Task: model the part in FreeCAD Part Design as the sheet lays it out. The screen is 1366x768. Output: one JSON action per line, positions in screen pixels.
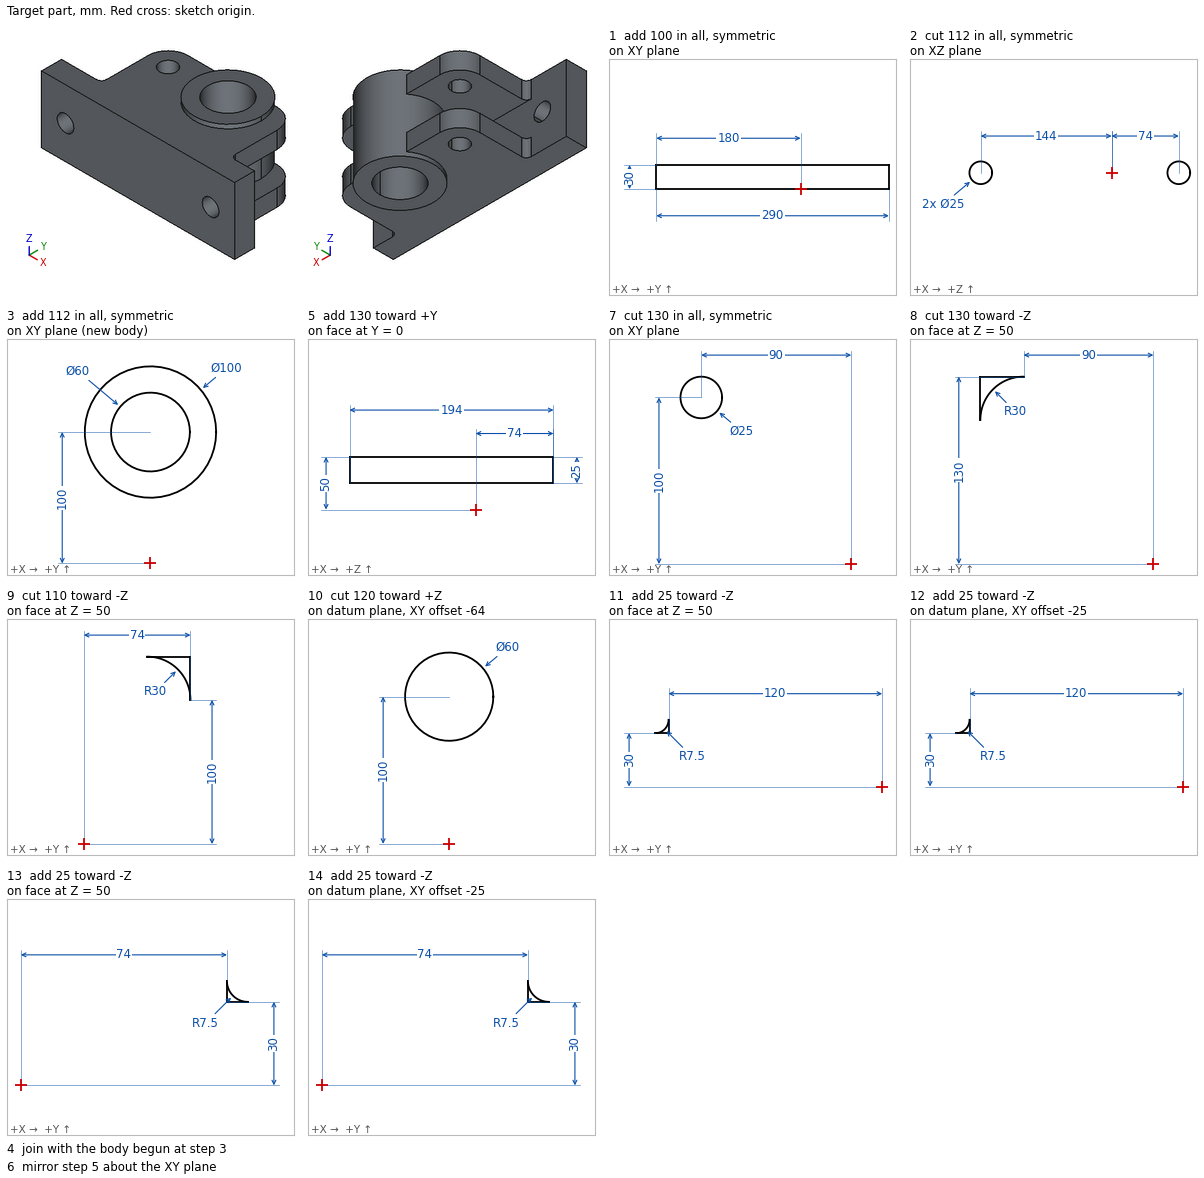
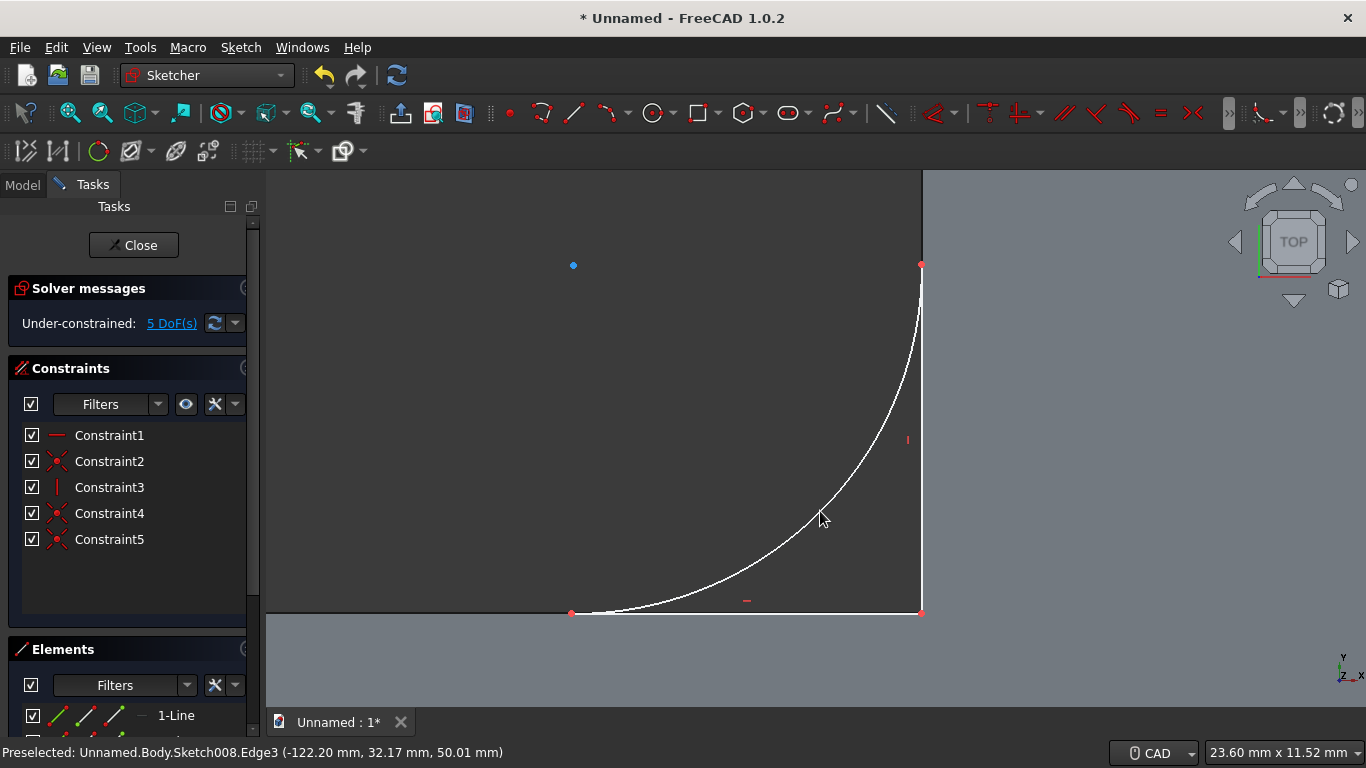
{"action": "left_click", "coordinate": [677, 614]}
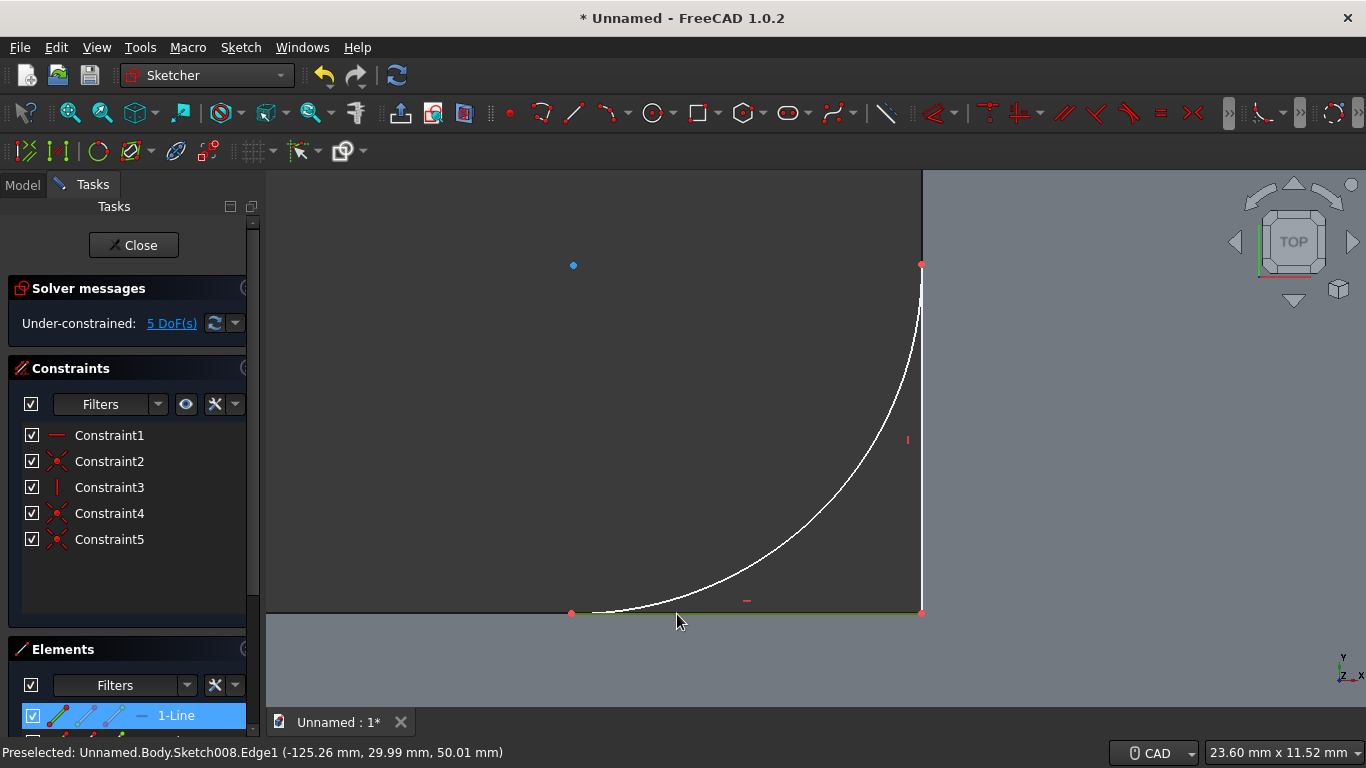
{"action": "left_click", "coordinate": [731, 576]}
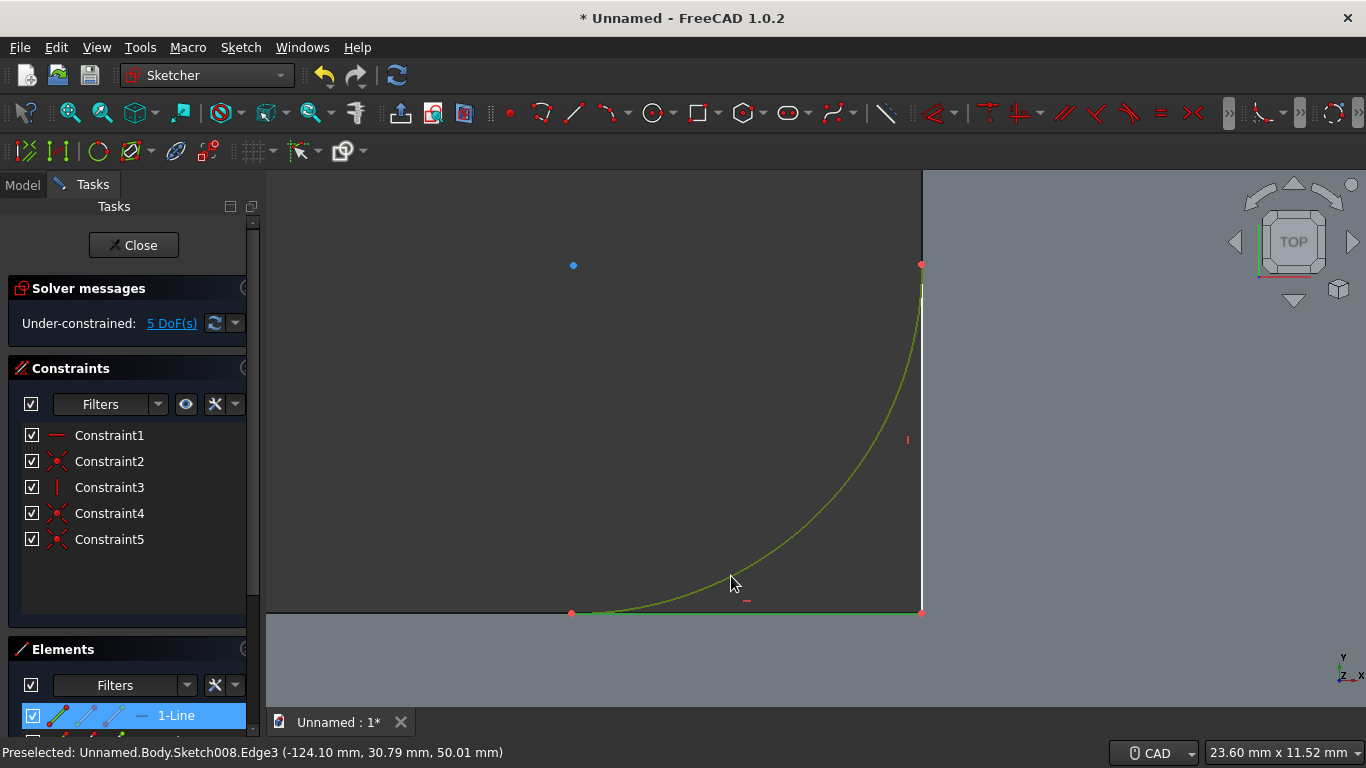
{"action": "left_click", "coordinate": [1130, 114]}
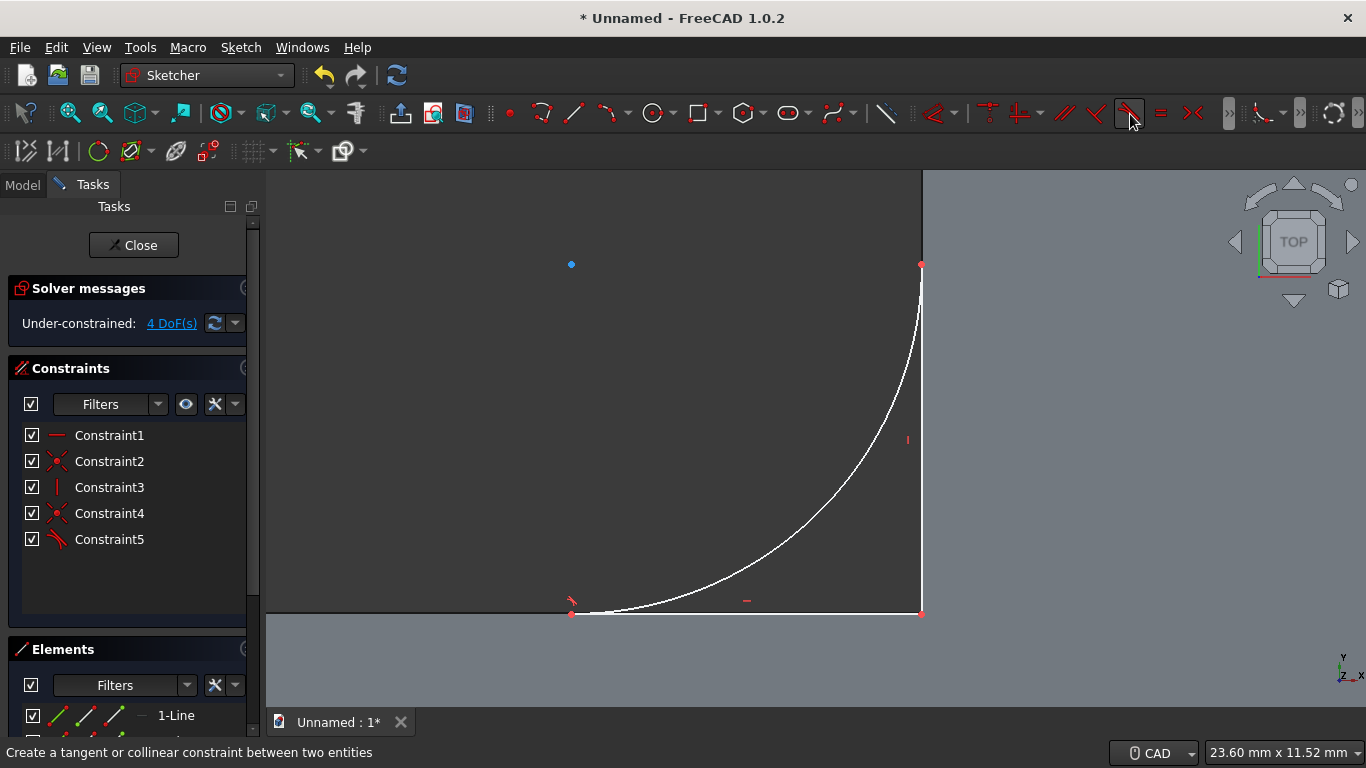
{"action": "left_click", "coordinate": [922, 509]}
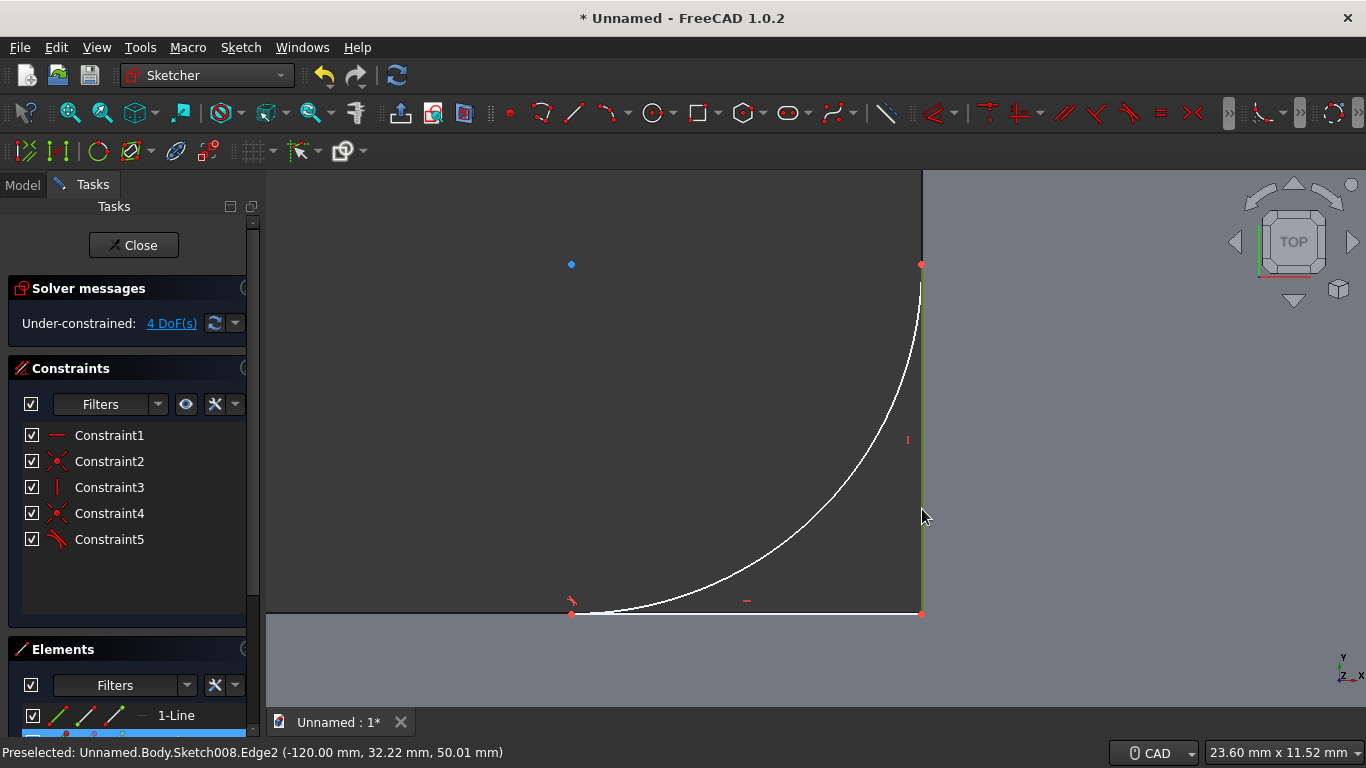
{"action": "left_click", "coordinate": [731, 576]}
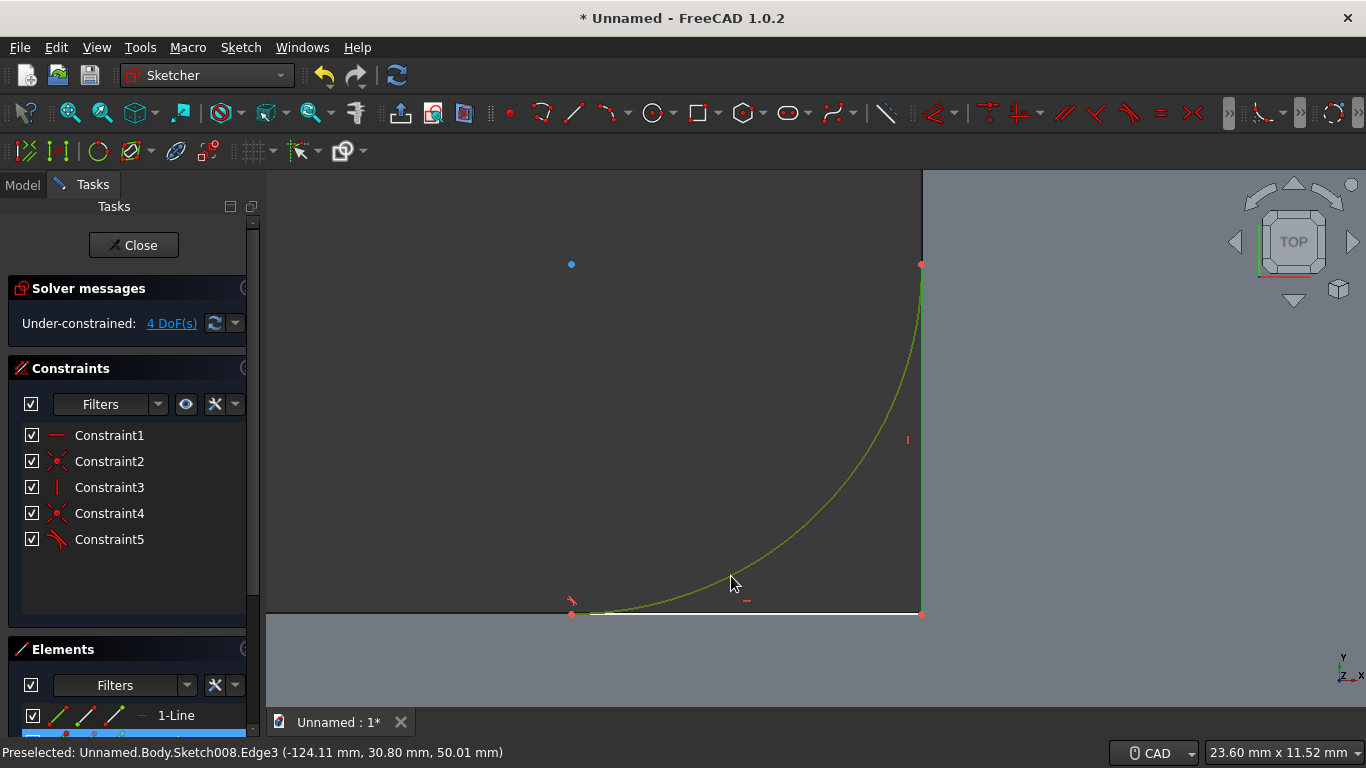
{"action": "left_click", "coordinate": [1130, 114]}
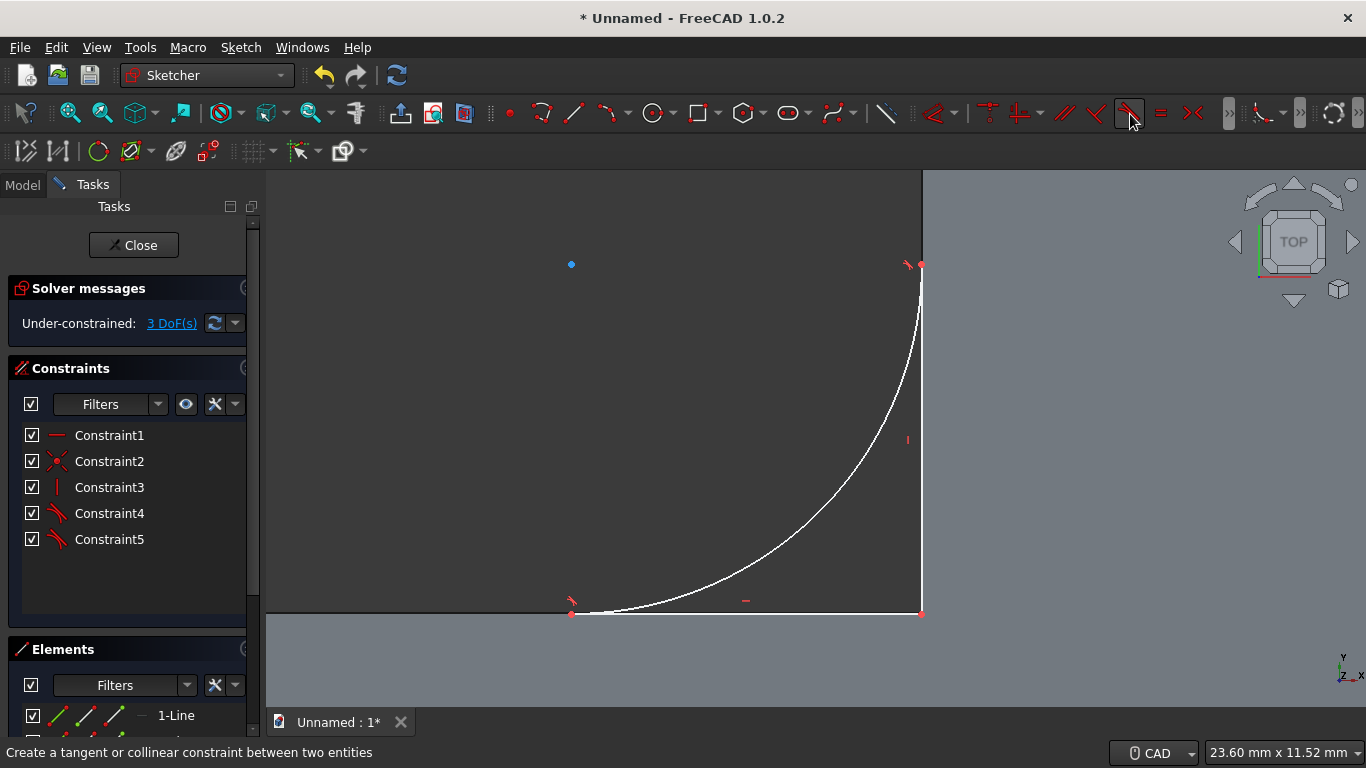
{"action": "left_click", "coordinate": [934, 114]}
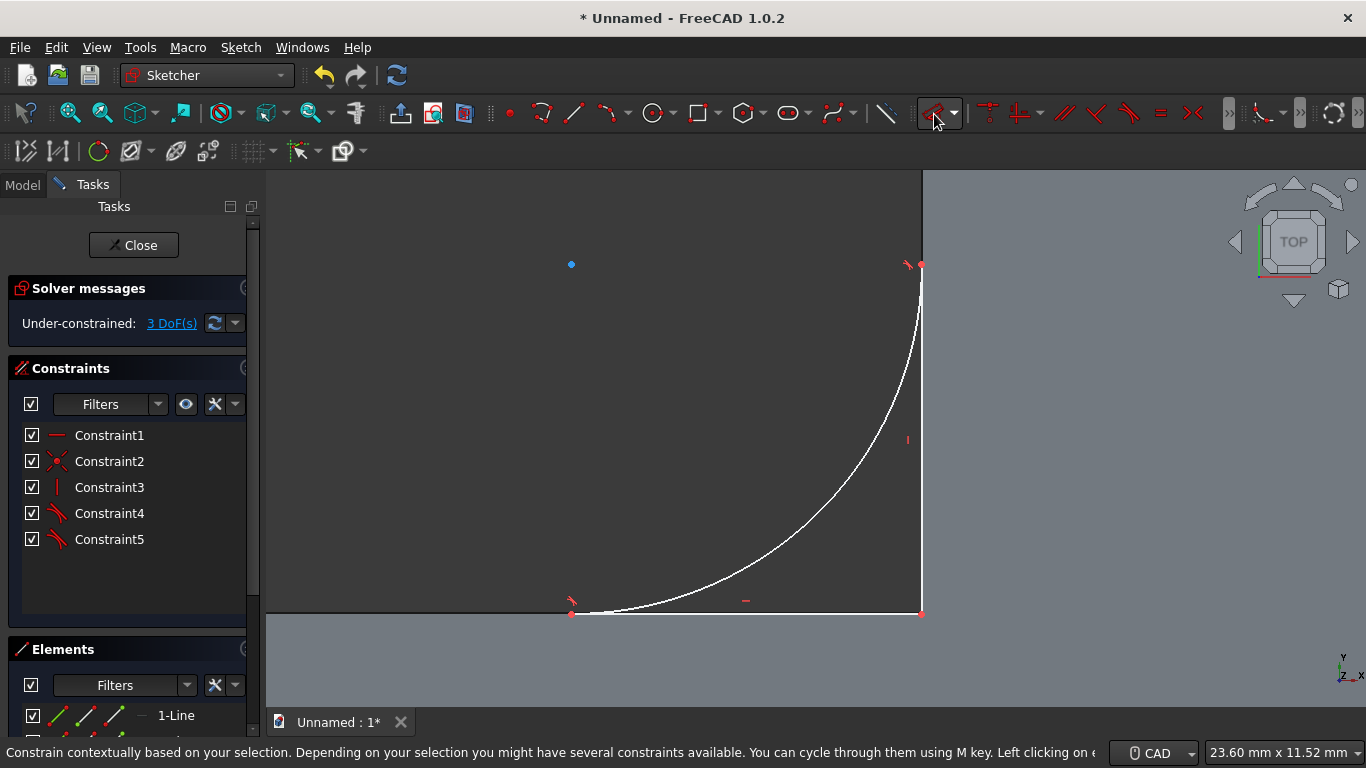
{"action": "left_click", "coordinate": [731, 576]}
{"action": "left_click", "coordinate": [561, 646]}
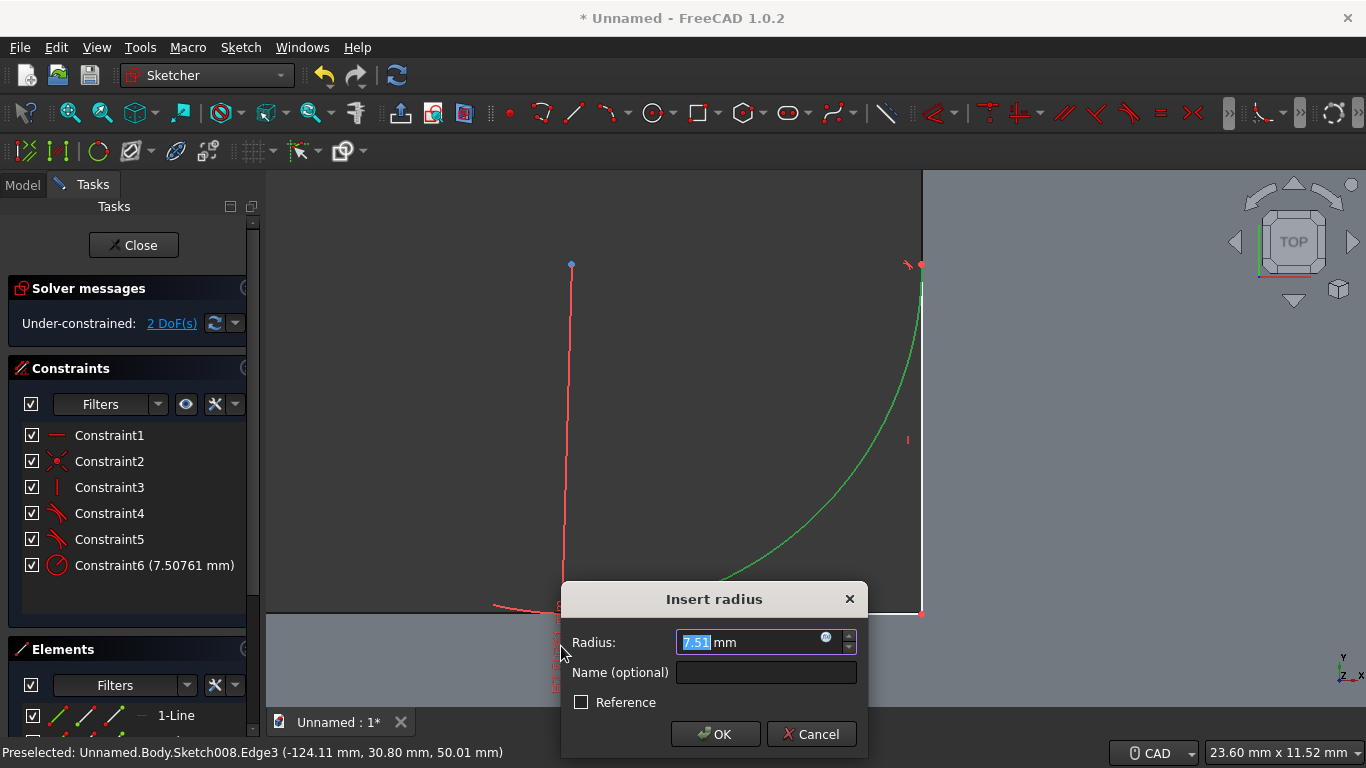
{"action": "type", "text": "7.5"}
{"action": "key", "text": "Return"}